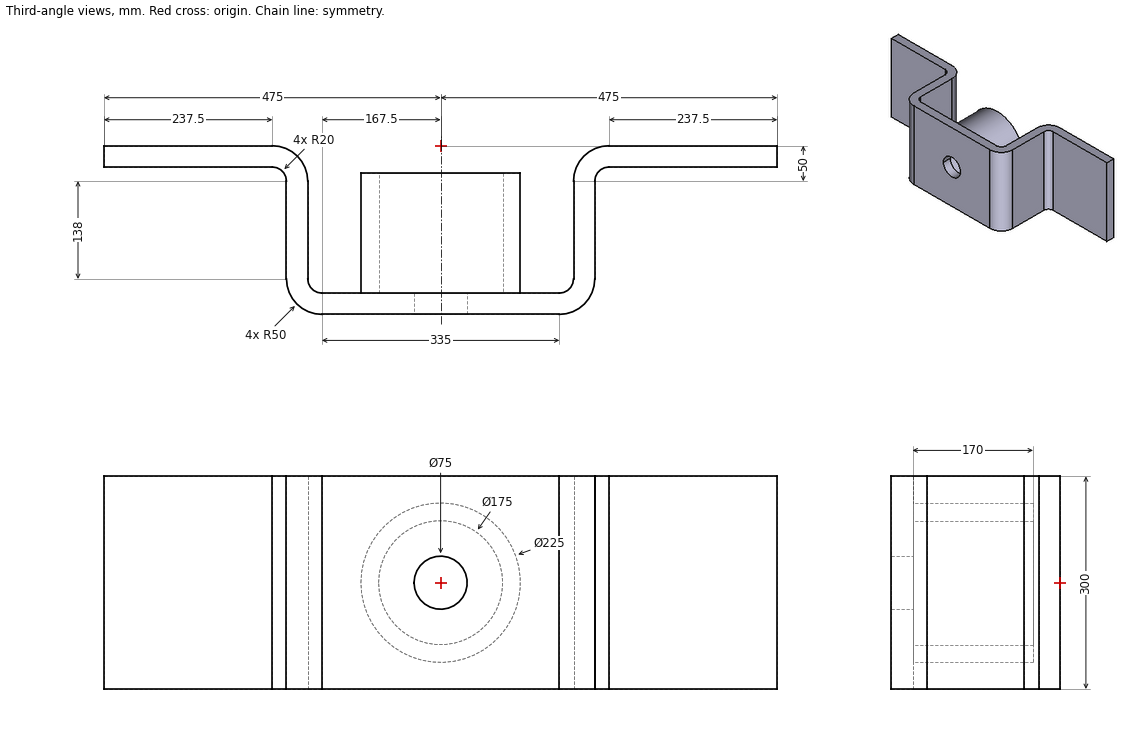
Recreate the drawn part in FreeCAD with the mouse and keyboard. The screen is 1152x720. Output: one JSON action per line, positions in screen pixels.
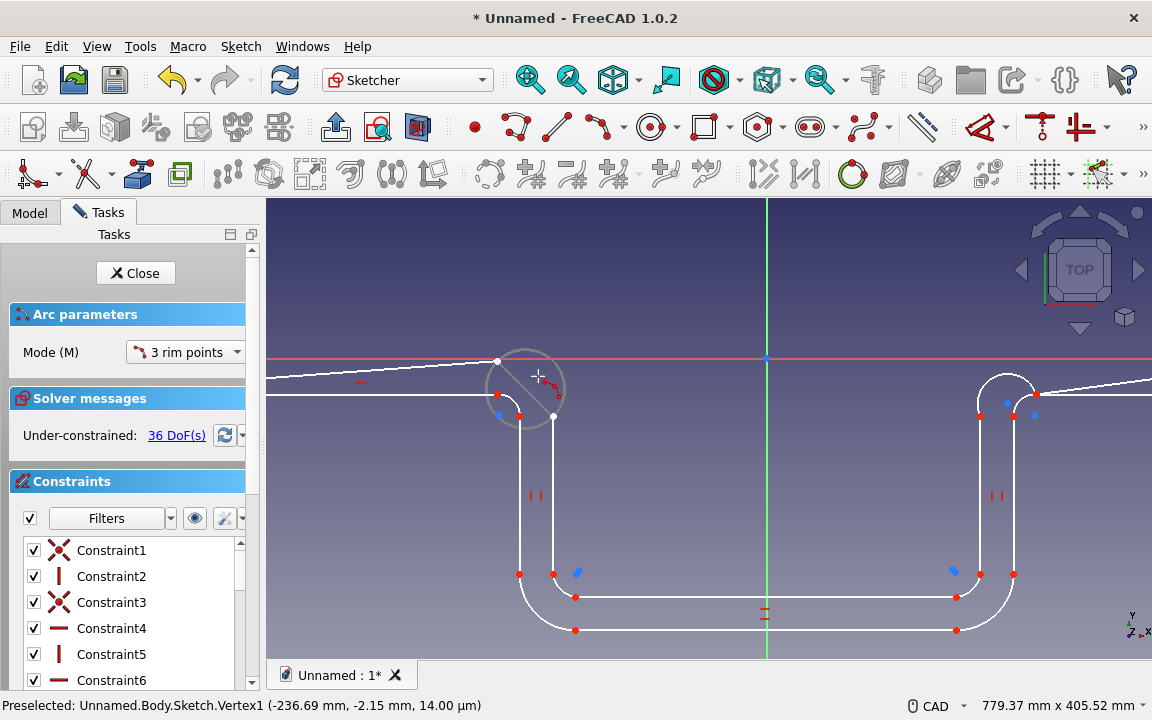
{"action": "left_click", "coordinate": [537, 375]}
{"action": "key", "text": "Escape"}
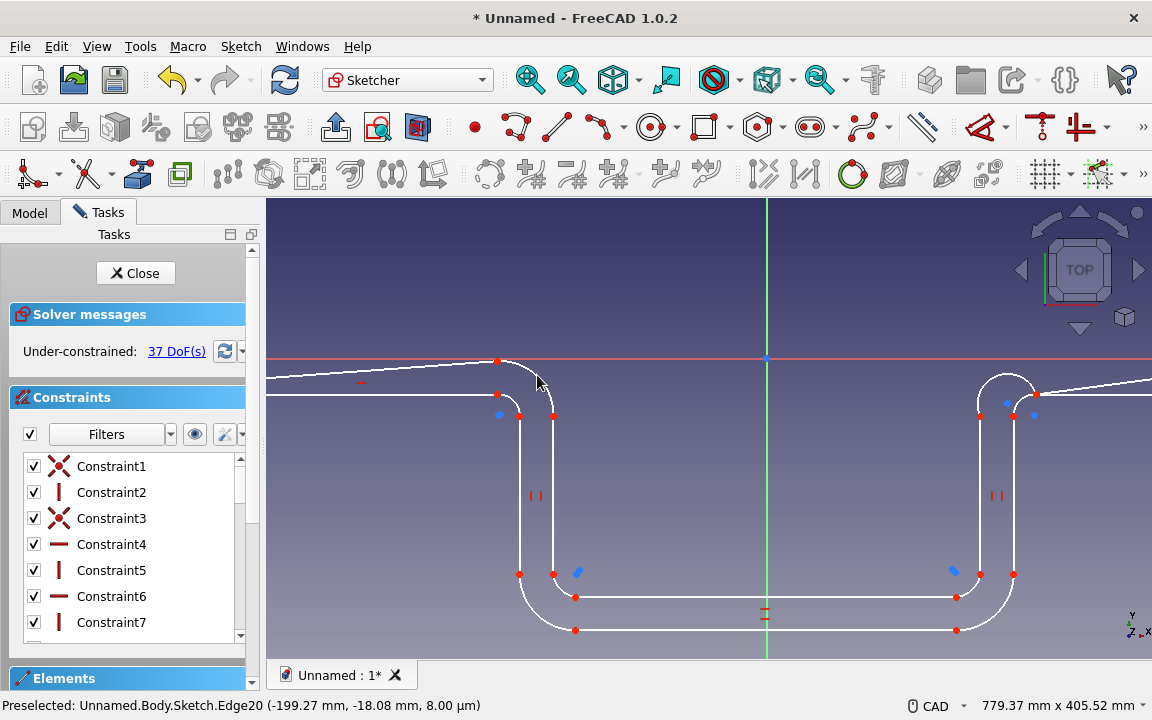
{"action": "left_click", "coordinate": [307, 395]}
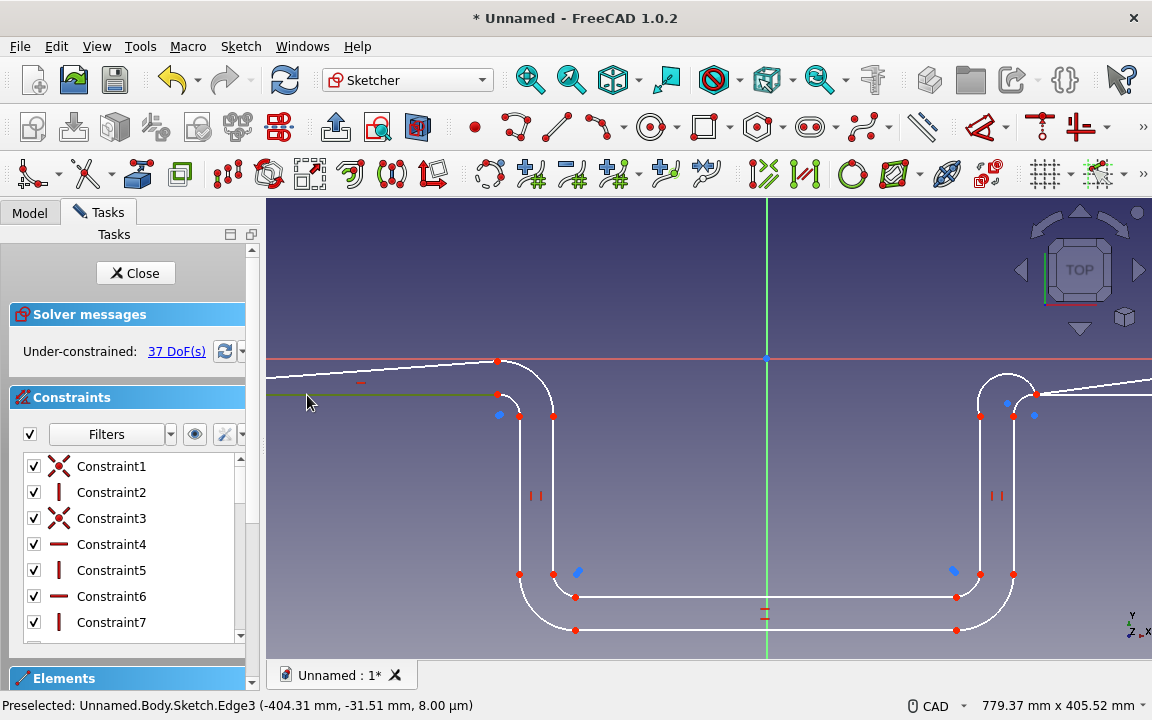
{"action": "scroll", "coordinate": [518, 406], "scroll_direction": "up", "scroll_amount": 2}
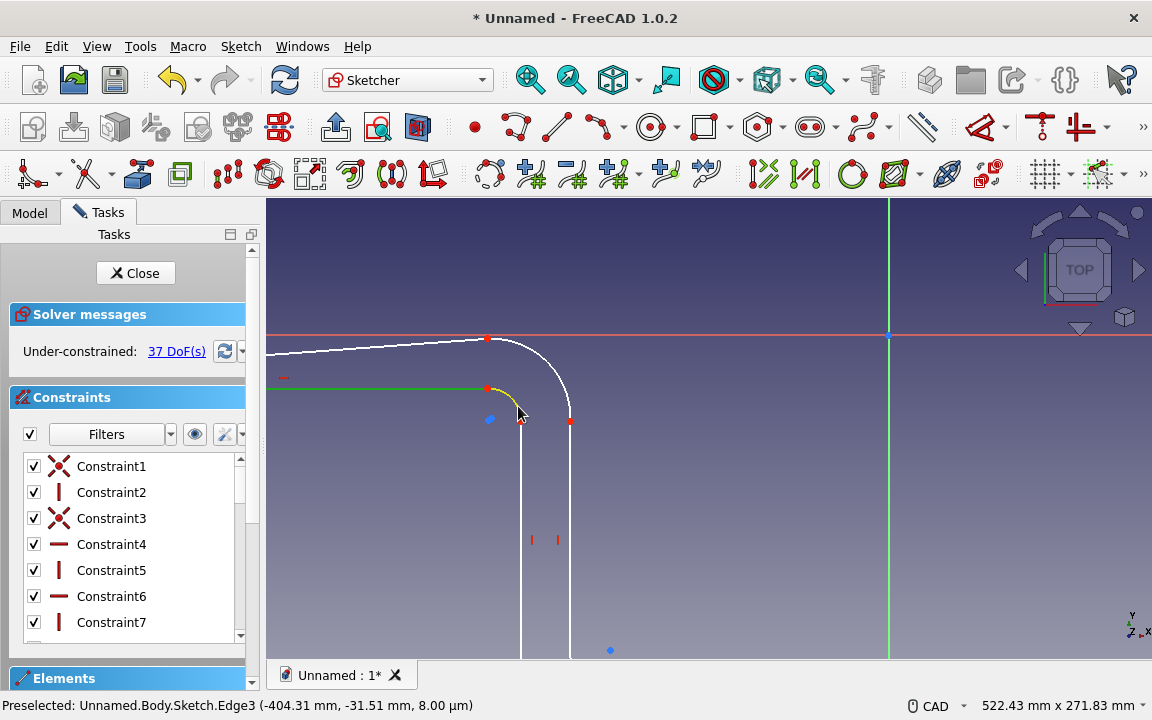
{"action": "left_click", "coordinate": [517, 406]}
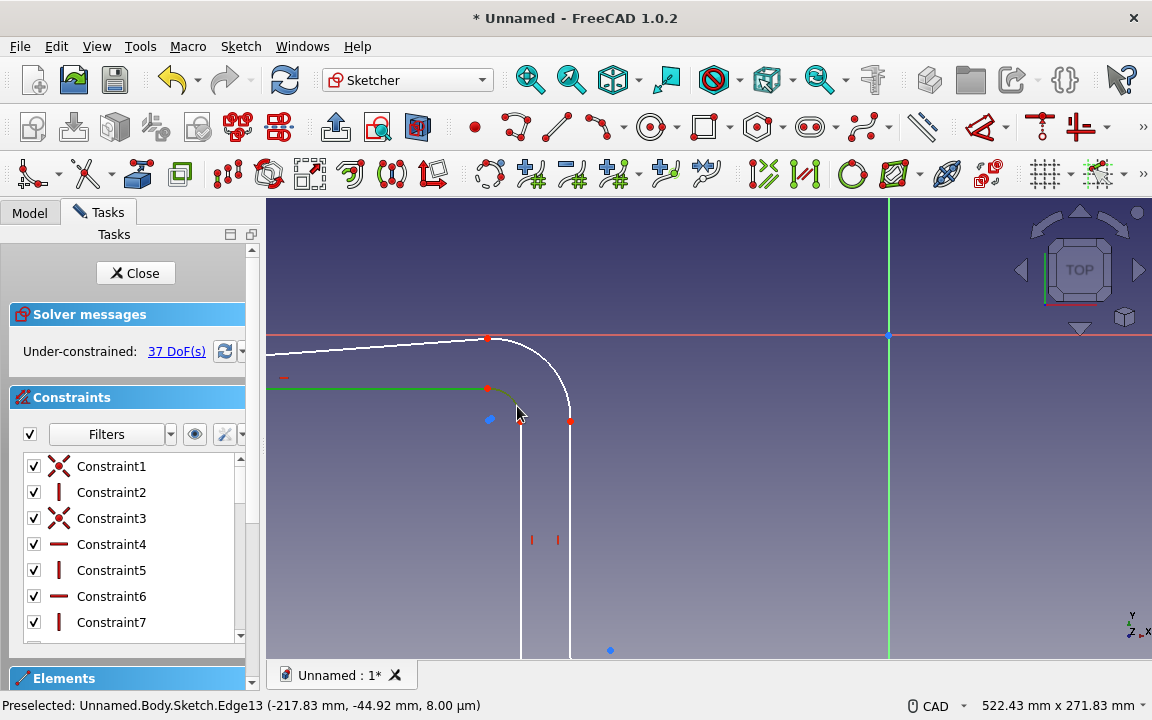
{"action": "key", "text": "t"}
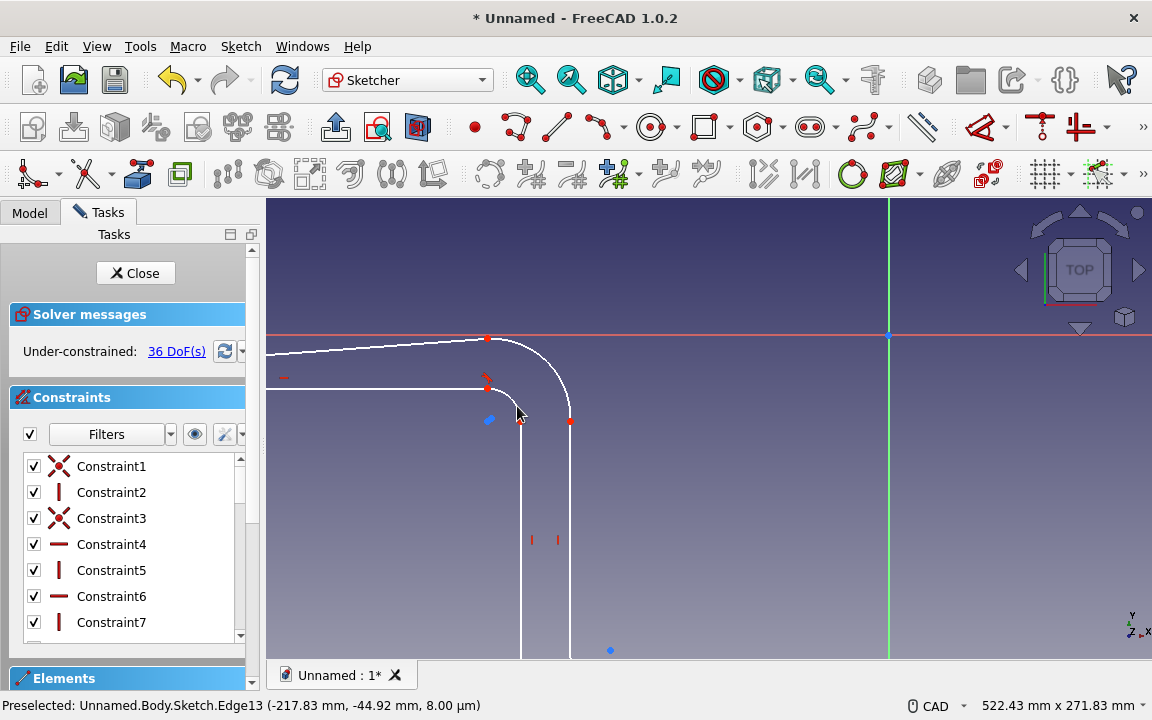
{"action": "left_click", "coordinate": [521, 493]}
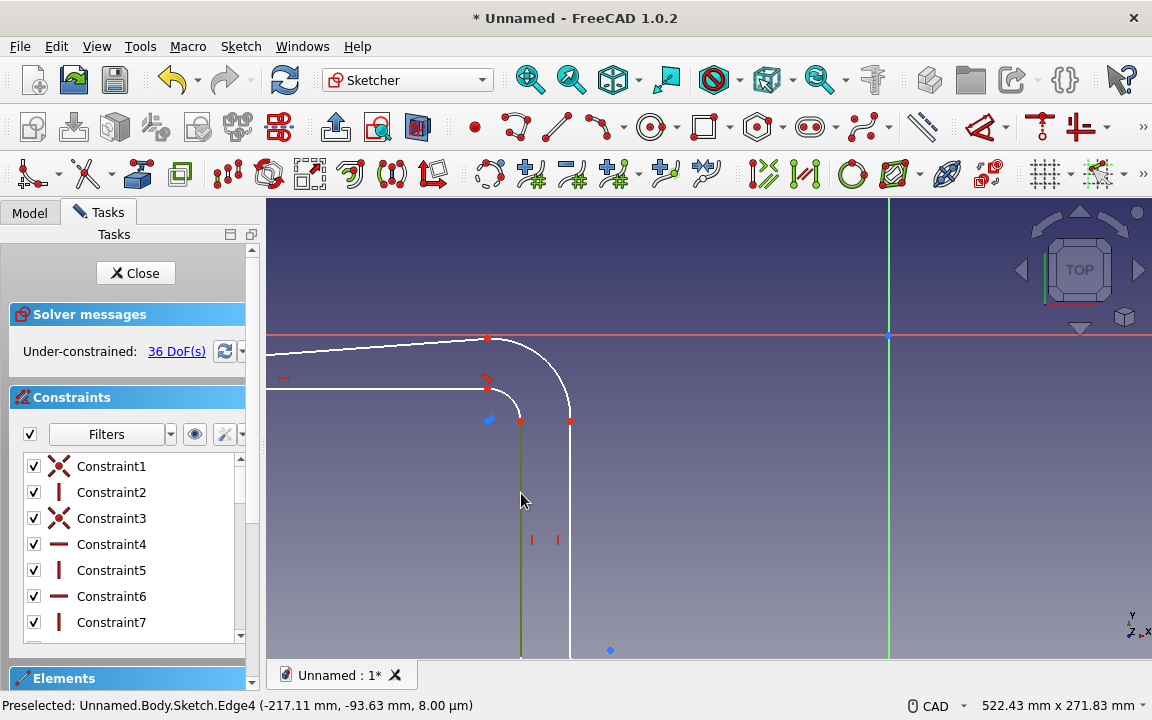
{"action": "left_click", "coordinate": [517, 407]}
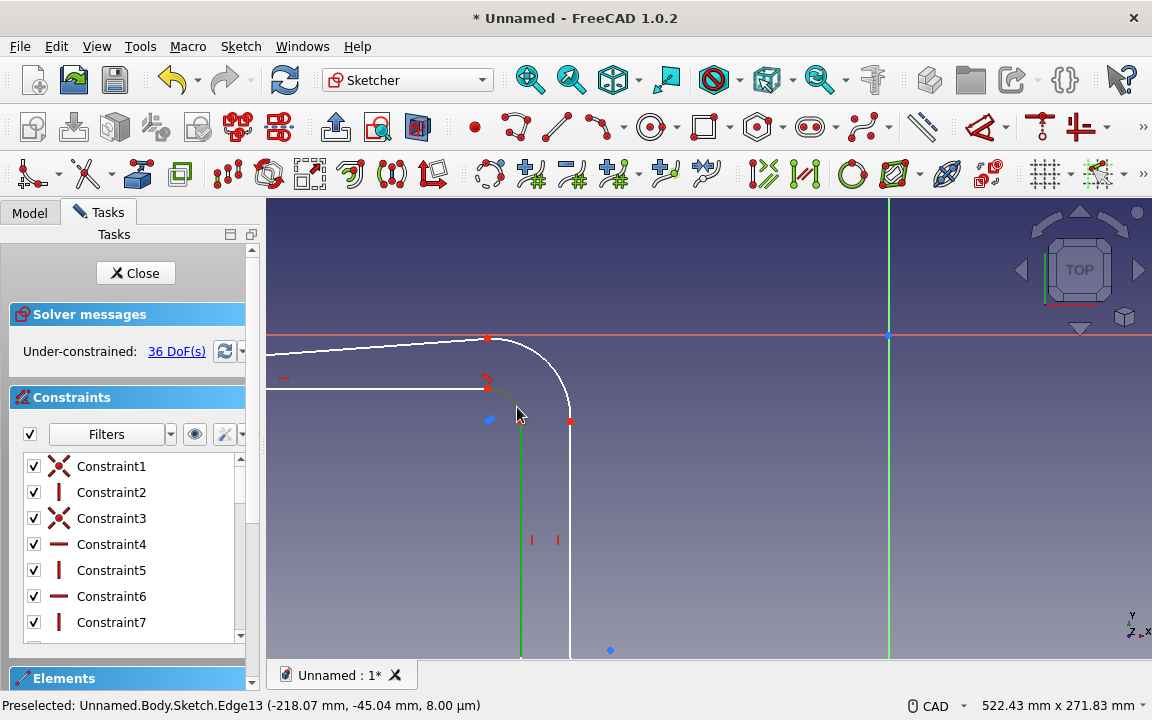
{"action": "key", "text": "t"}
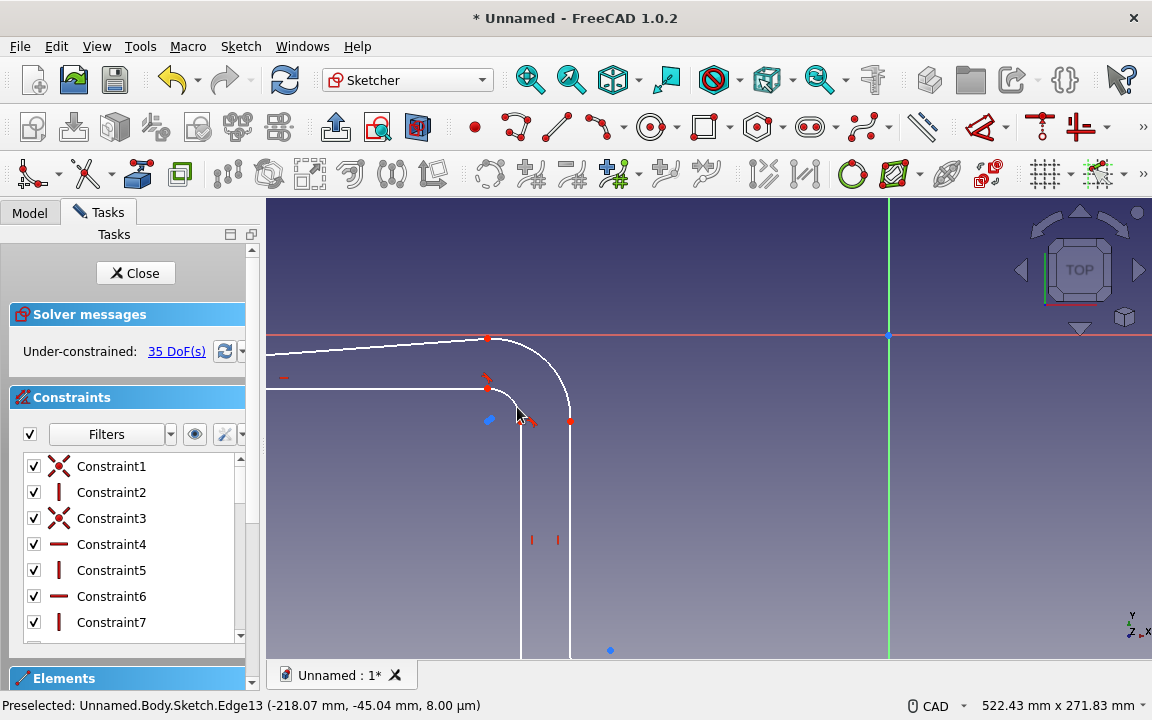
{"action": "scroll", "coordinate": [533, 382], "scroll_direction": "down", "scroll_amount": 6}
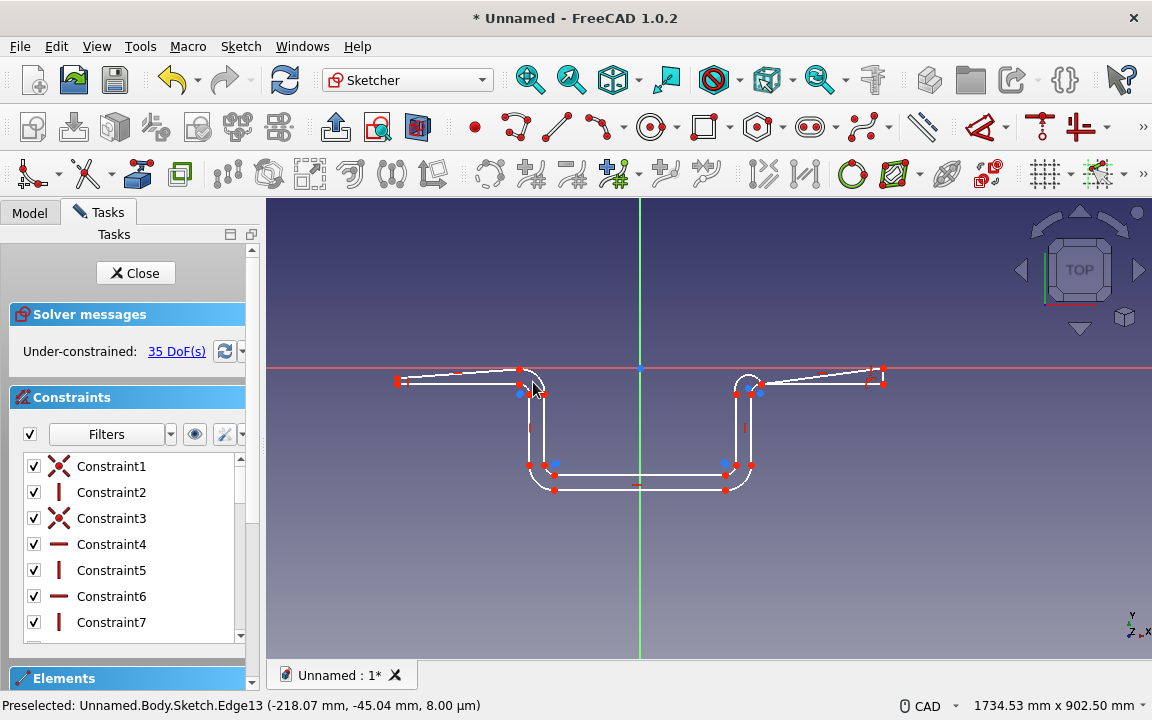
{"action": "left_click", "coordinate": [751, 444]}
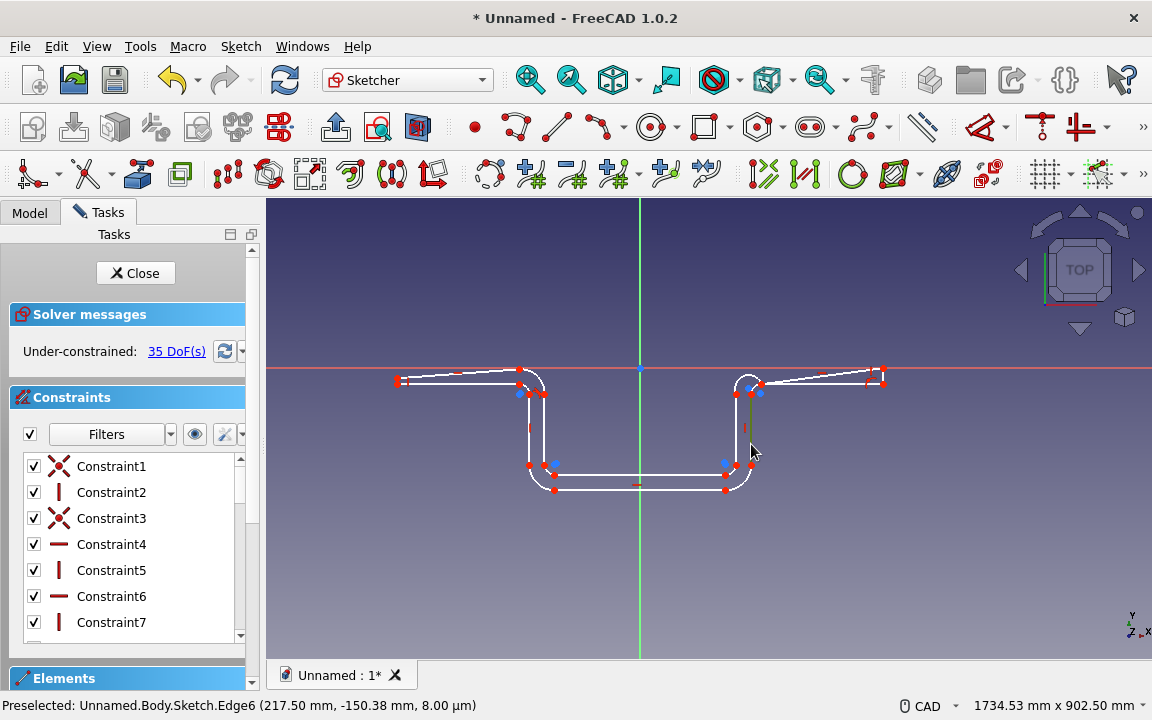
{"action": "scroll", "coordinate": [754, 387], "scroll_direction": "up", "scroll_amount": 3}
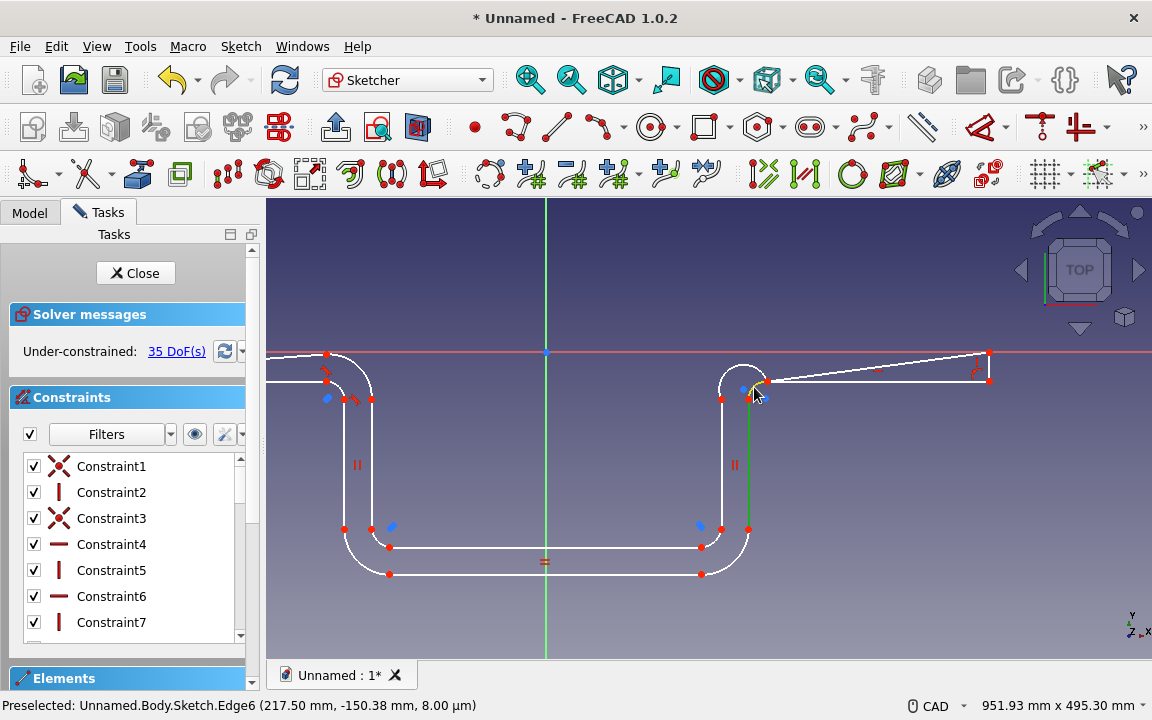
{"action": "left_click", "coordinate": [754, 387]}